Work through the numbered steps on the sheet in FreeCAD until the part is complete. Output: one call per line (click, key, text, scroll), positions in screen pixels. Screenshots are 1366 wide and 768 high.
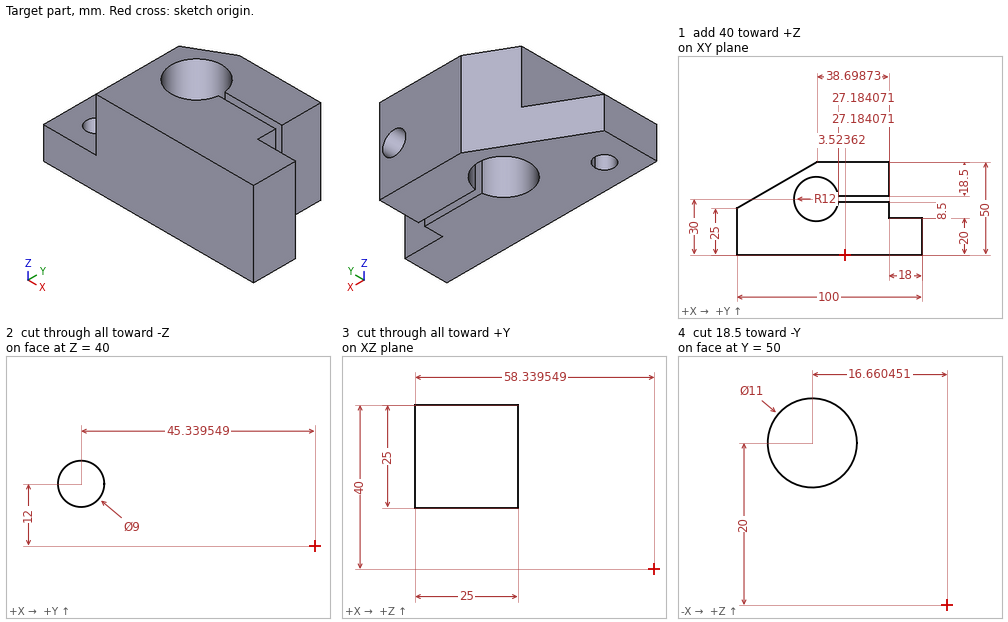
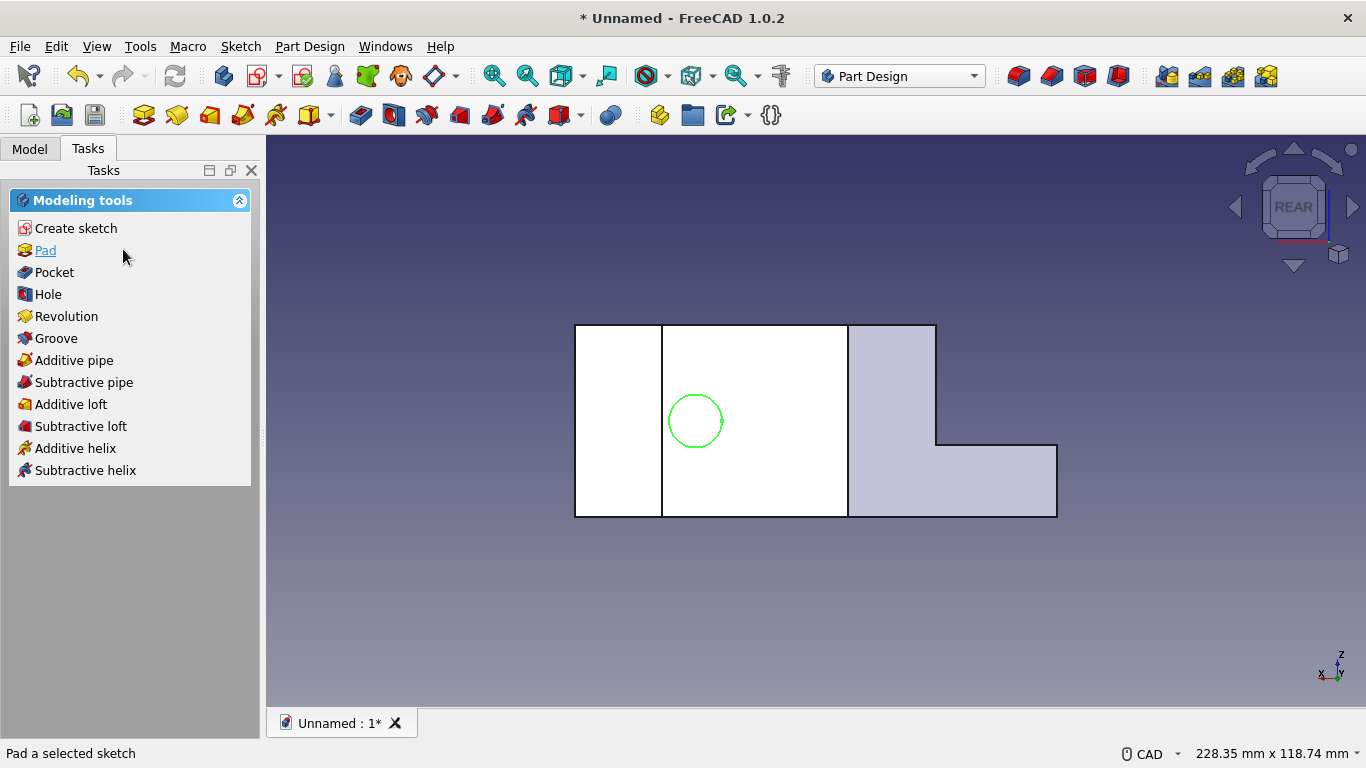
click(361, 116)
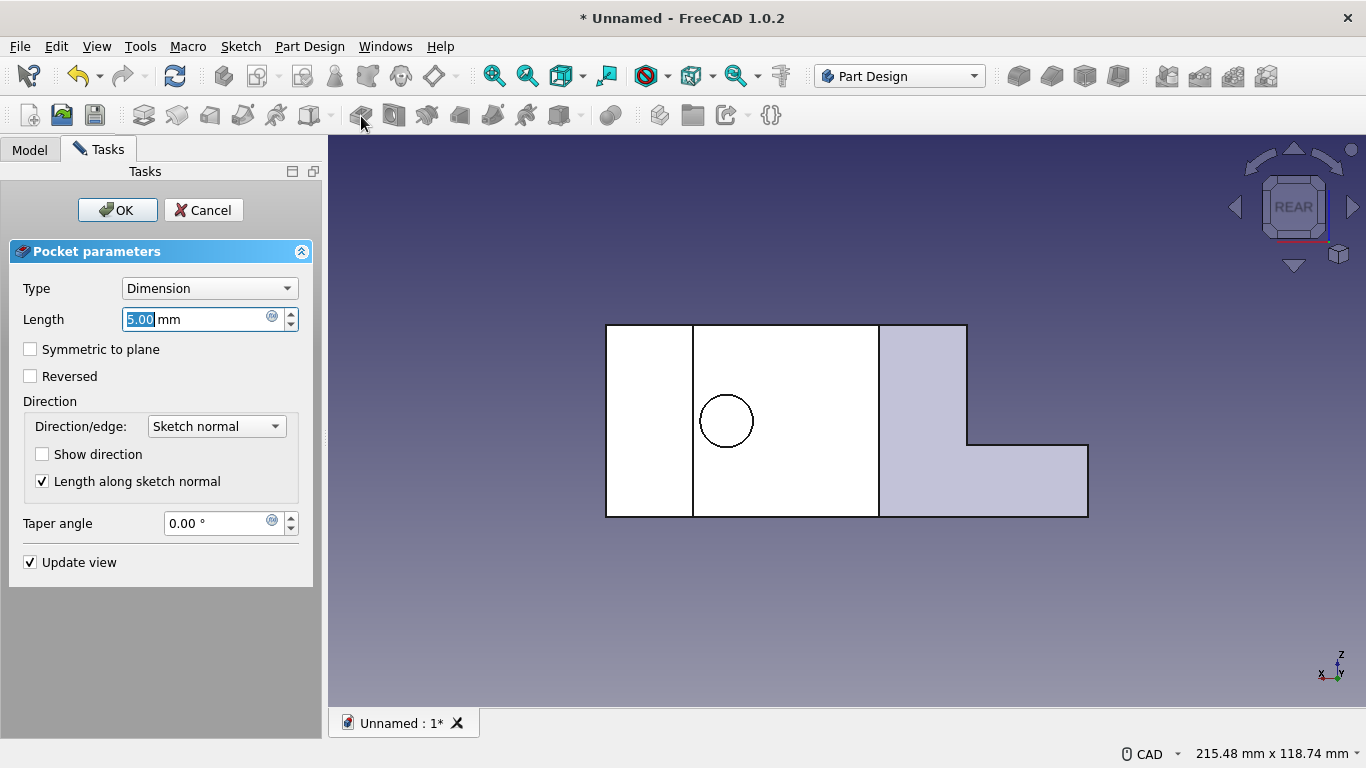
text(18.5)
key(Tab)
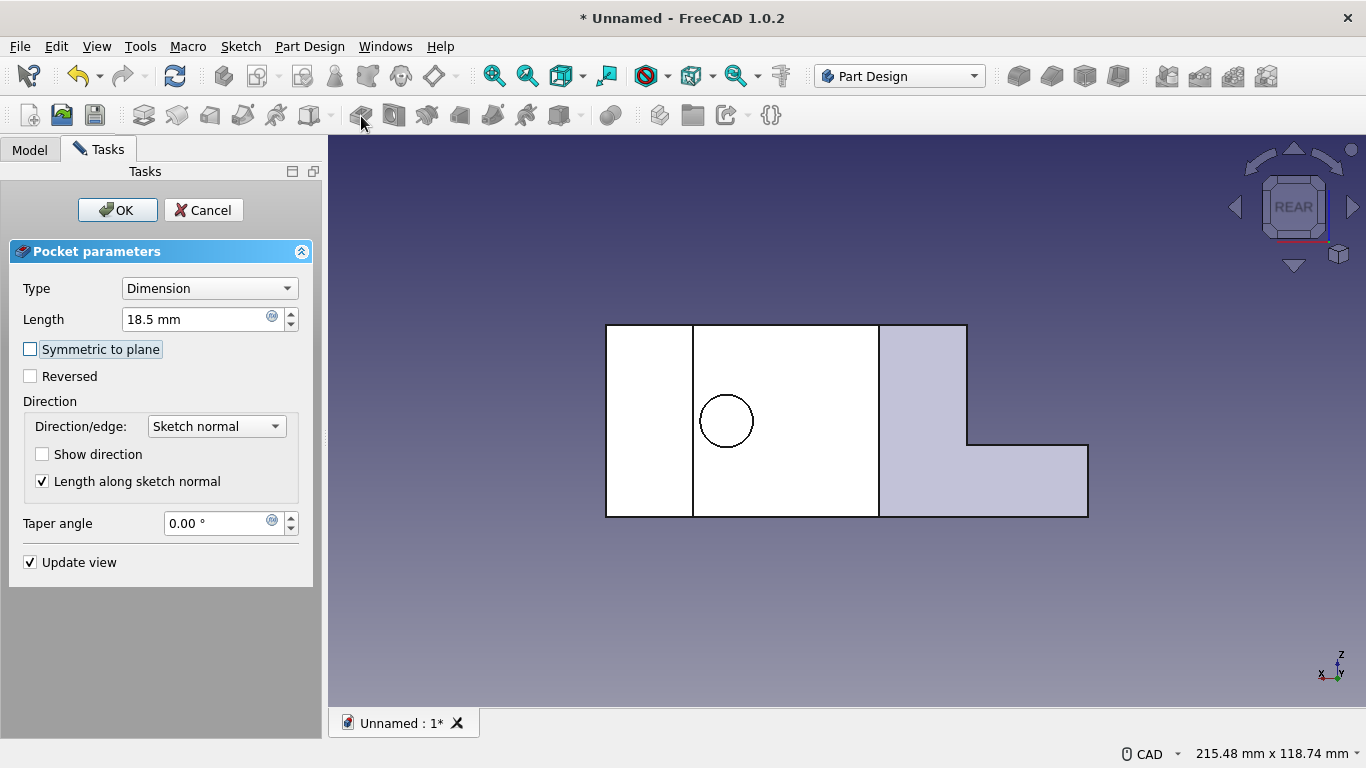
click(118, 210)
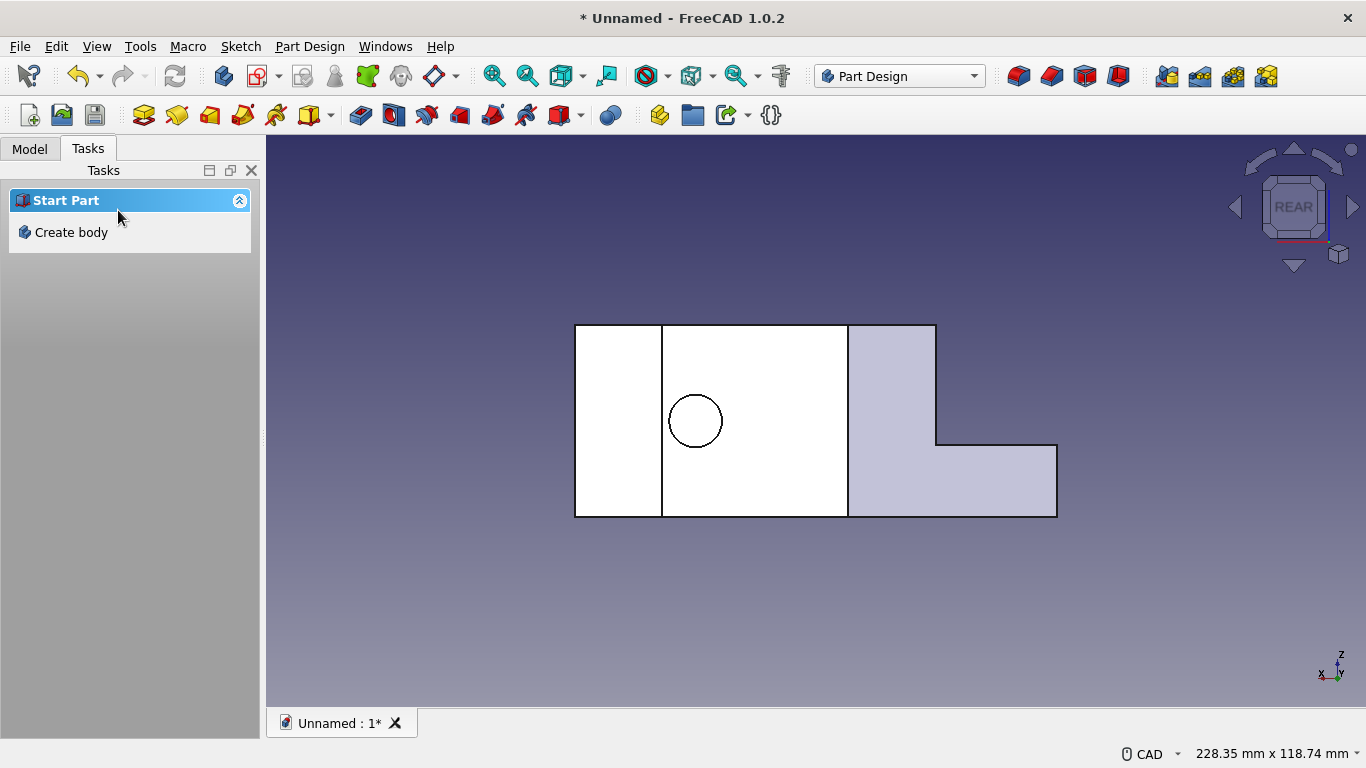
key(0)